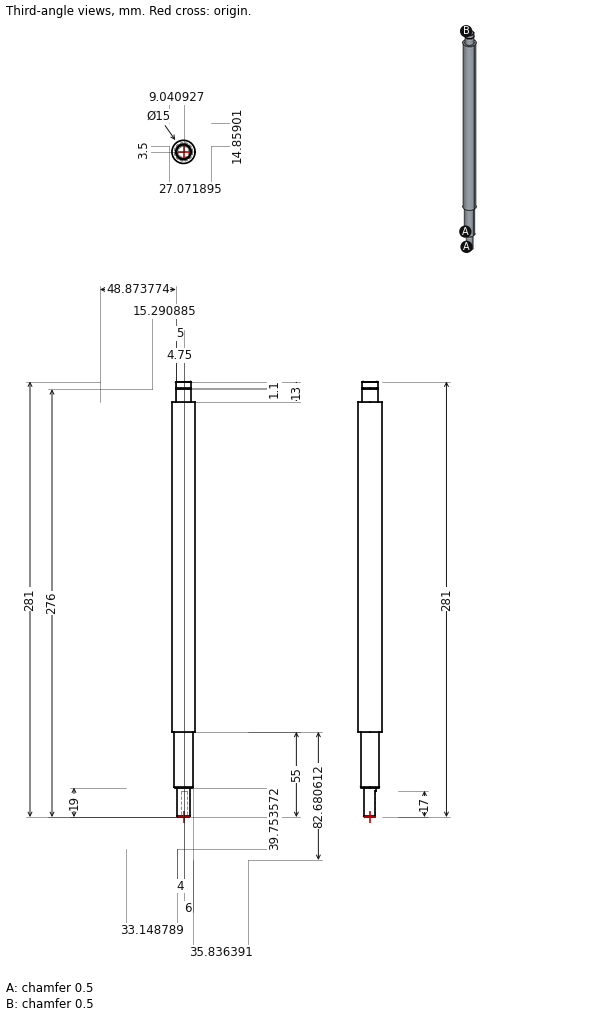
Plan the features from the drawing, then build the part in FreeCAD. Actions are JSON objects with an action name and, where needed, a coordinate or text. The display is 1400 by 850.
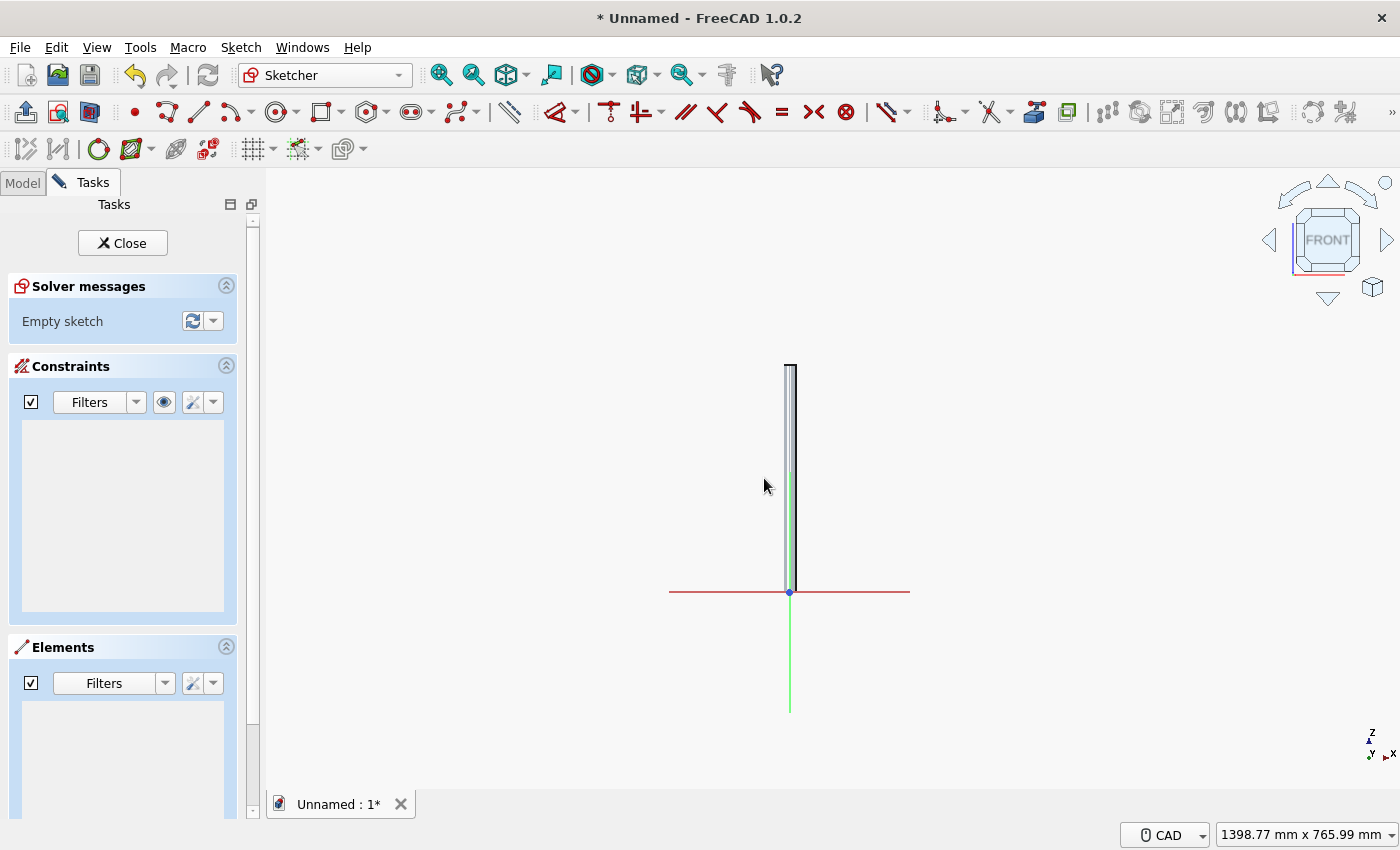
{"action": "scroll", "coordinate": [766, 363], "scroll_direction": "up", "scroll_amount": 14}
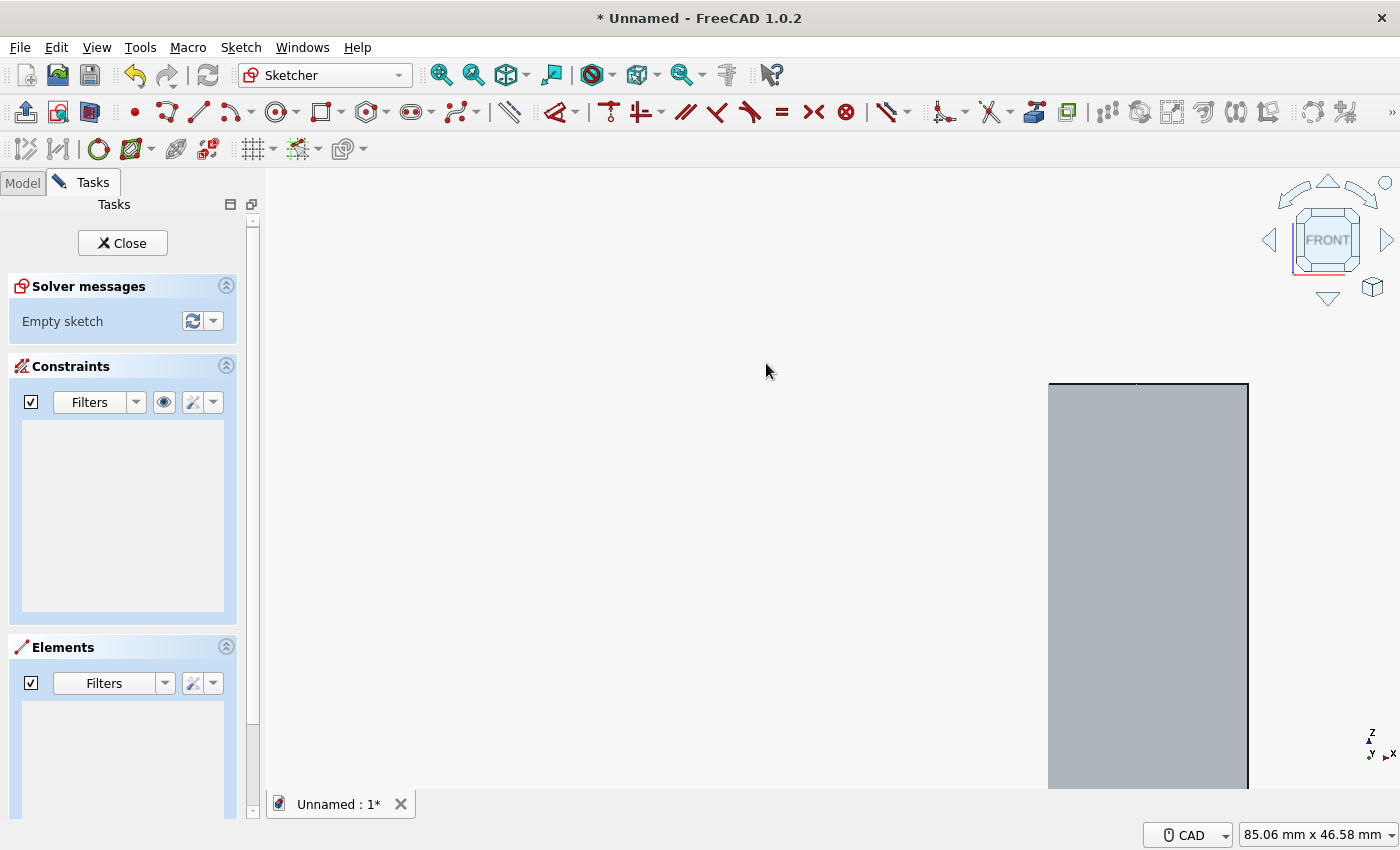
{"action": "left_click", "coordinate": [322, 112]}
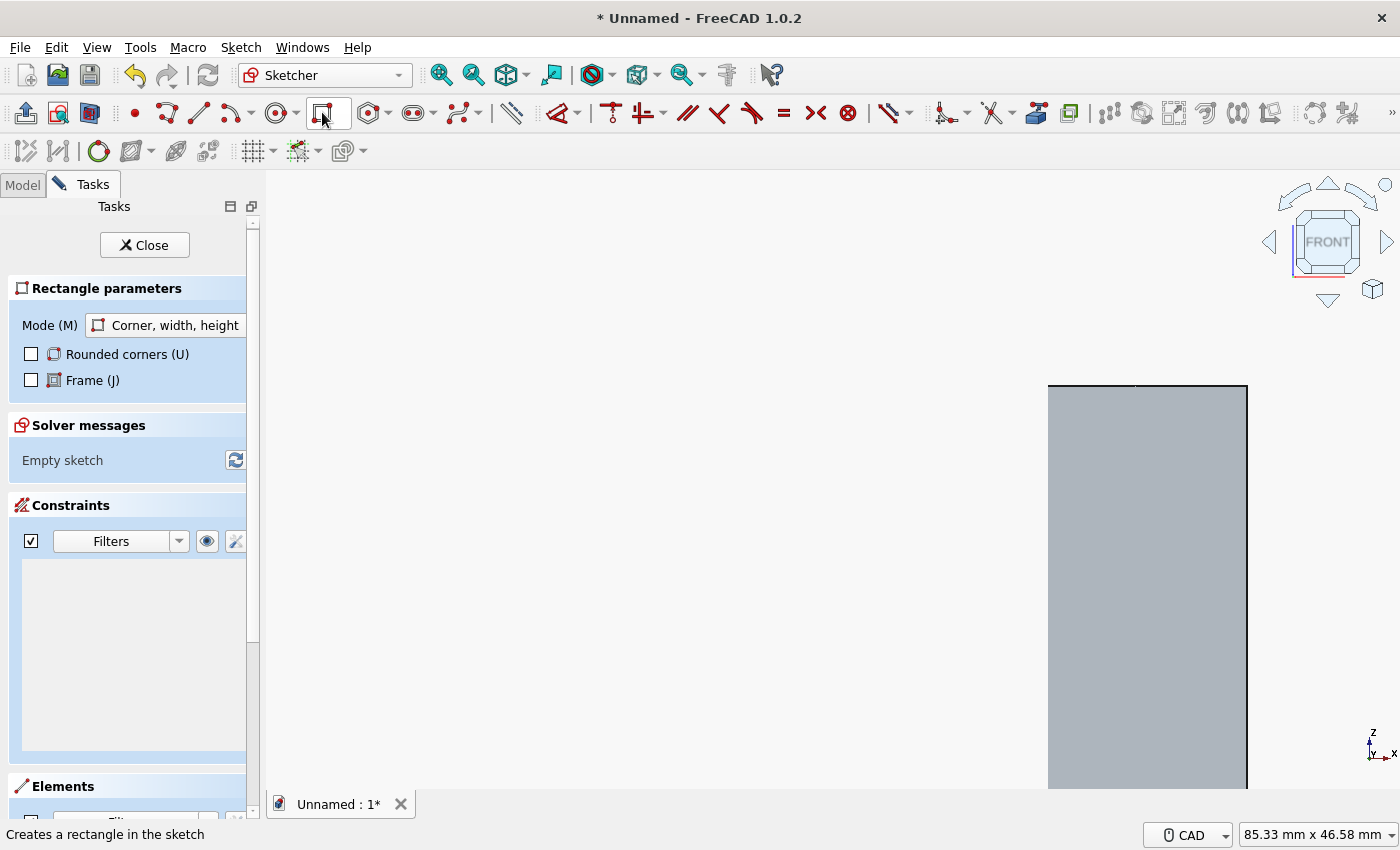
{"action": "left_click", "coordinate": [431, 386]}
{"action": "mouse_move", "coordinate": [1081, 558]}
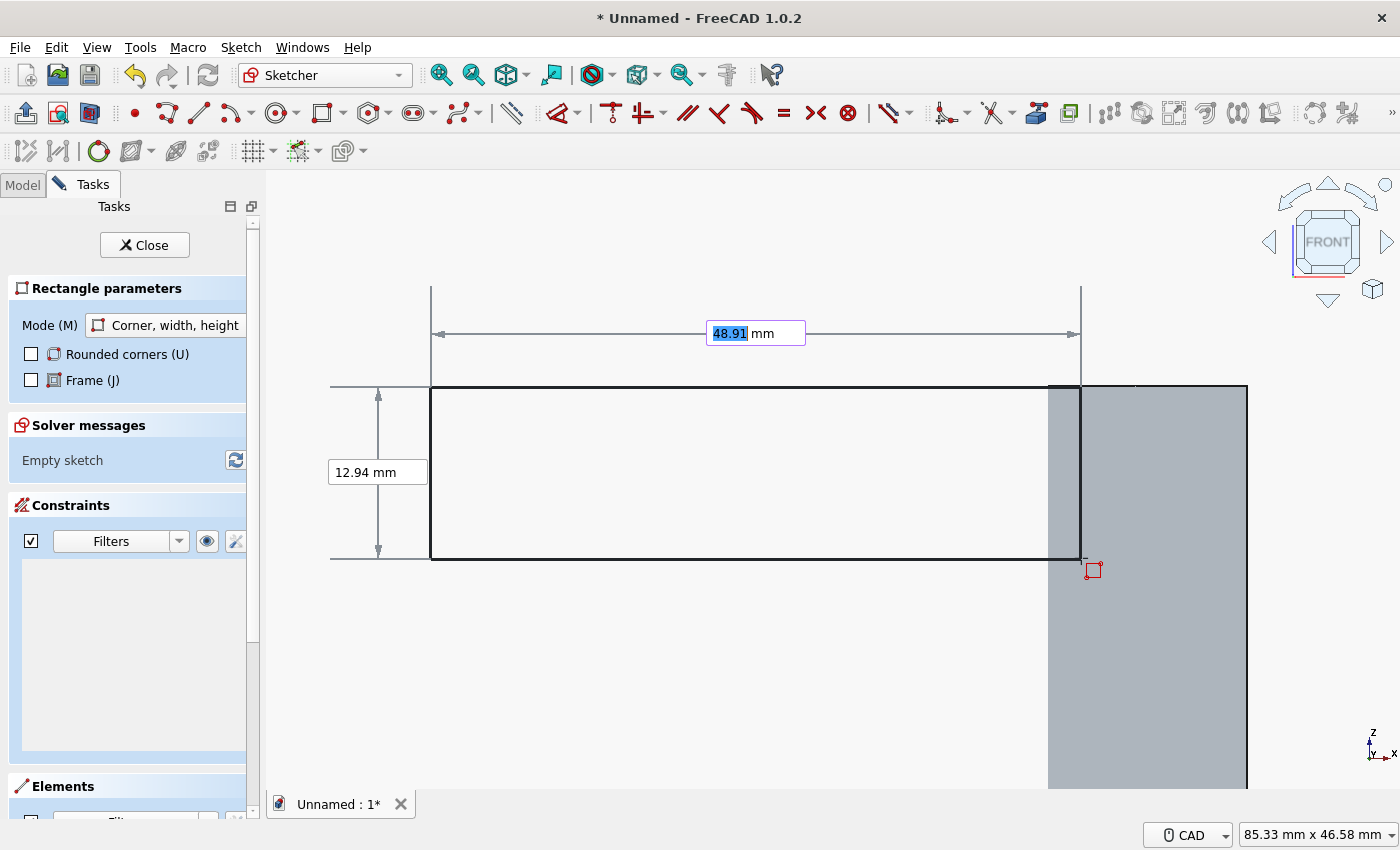
{"action": "type", "text": "48.873774"}
{"action": "key", "text": "Tab"}
{"action": "type", "text": "13"}
{"action": "key", "text": "Return"}
{"action": "key", "text": "Escape"}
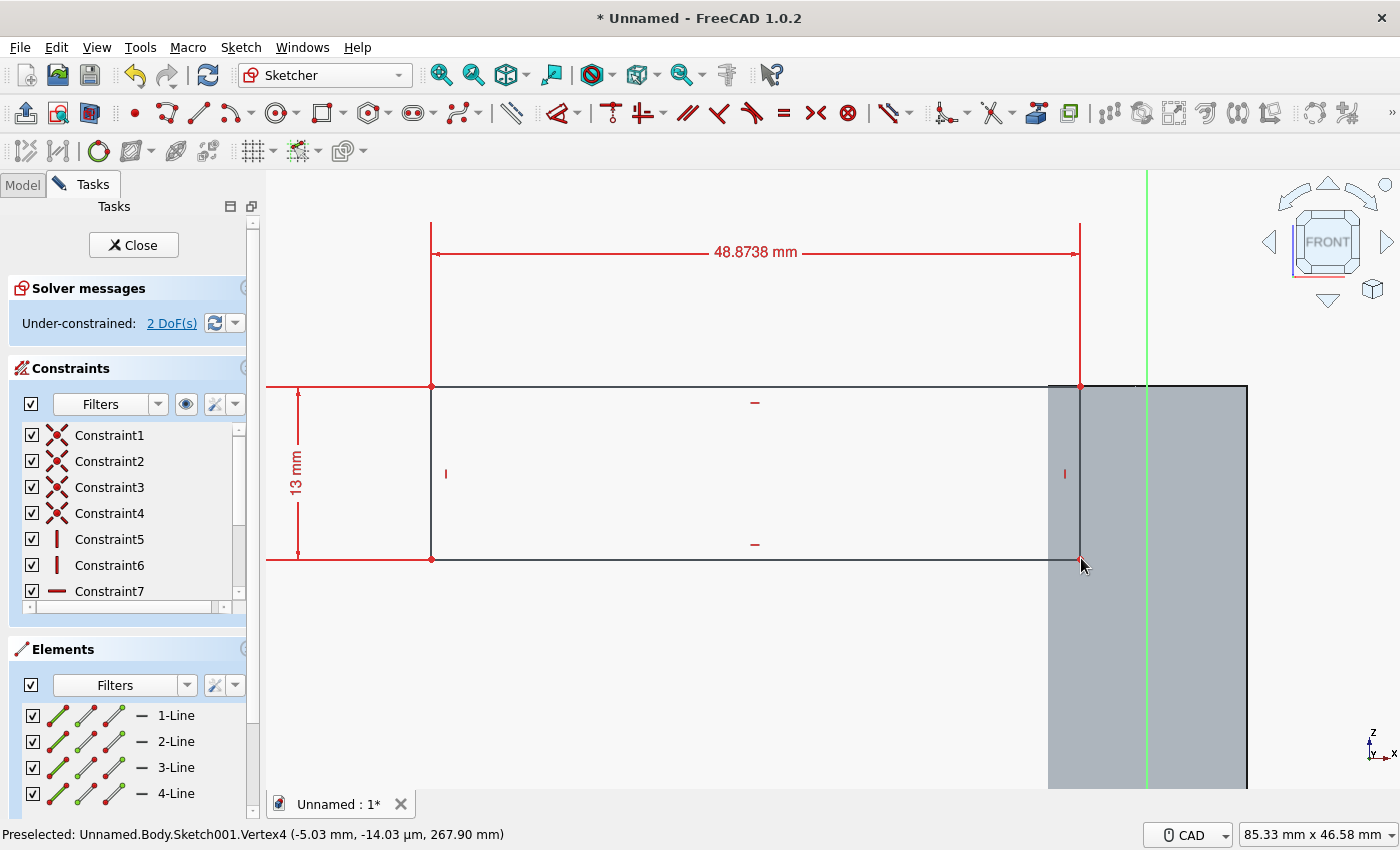
{"action": "left_click", "coordinate": [558, 114]}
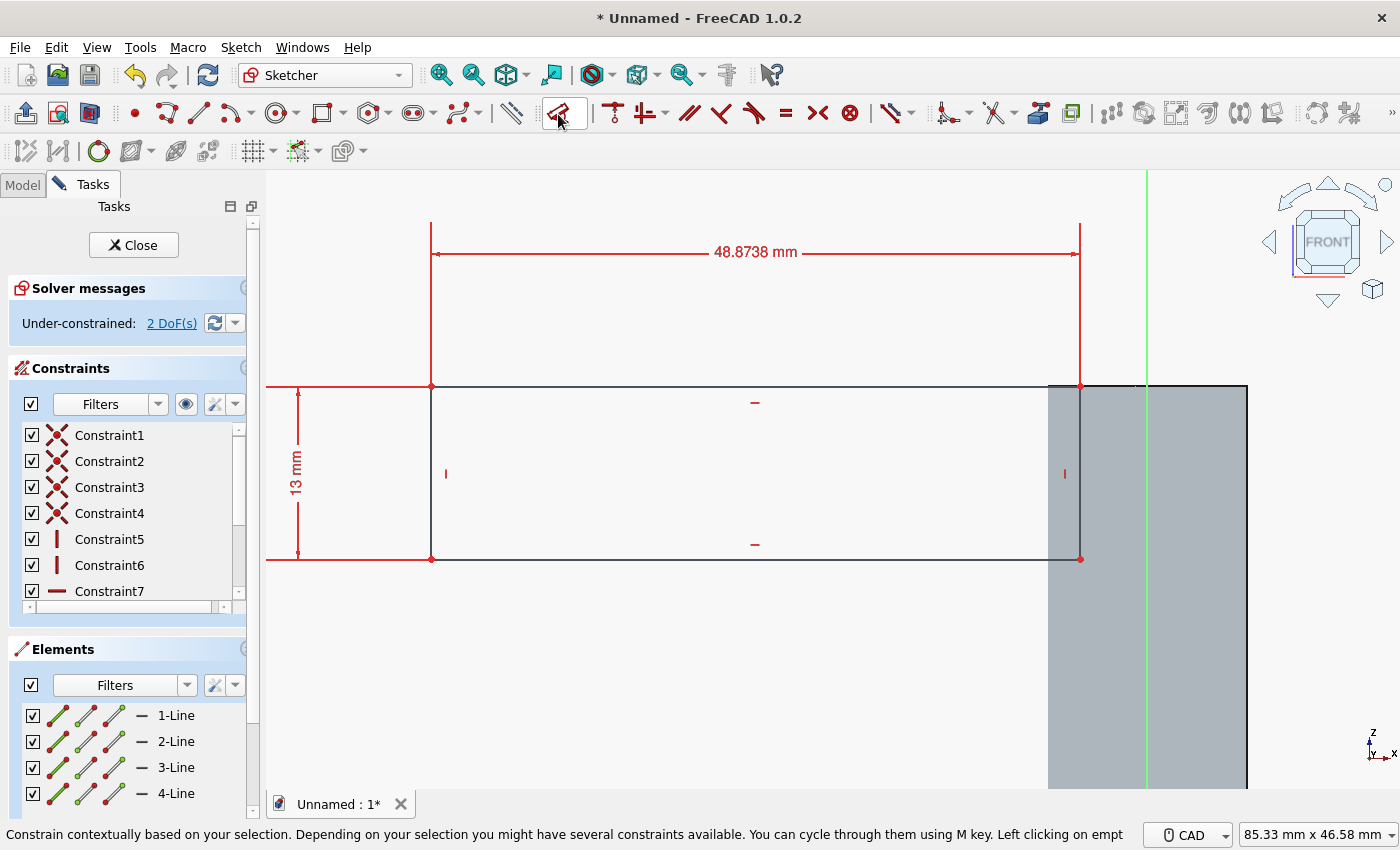
{"action": "left_click", "coordinate": [1080, 560]}
{"action": "left_click", "coordinate": [1114, 526]}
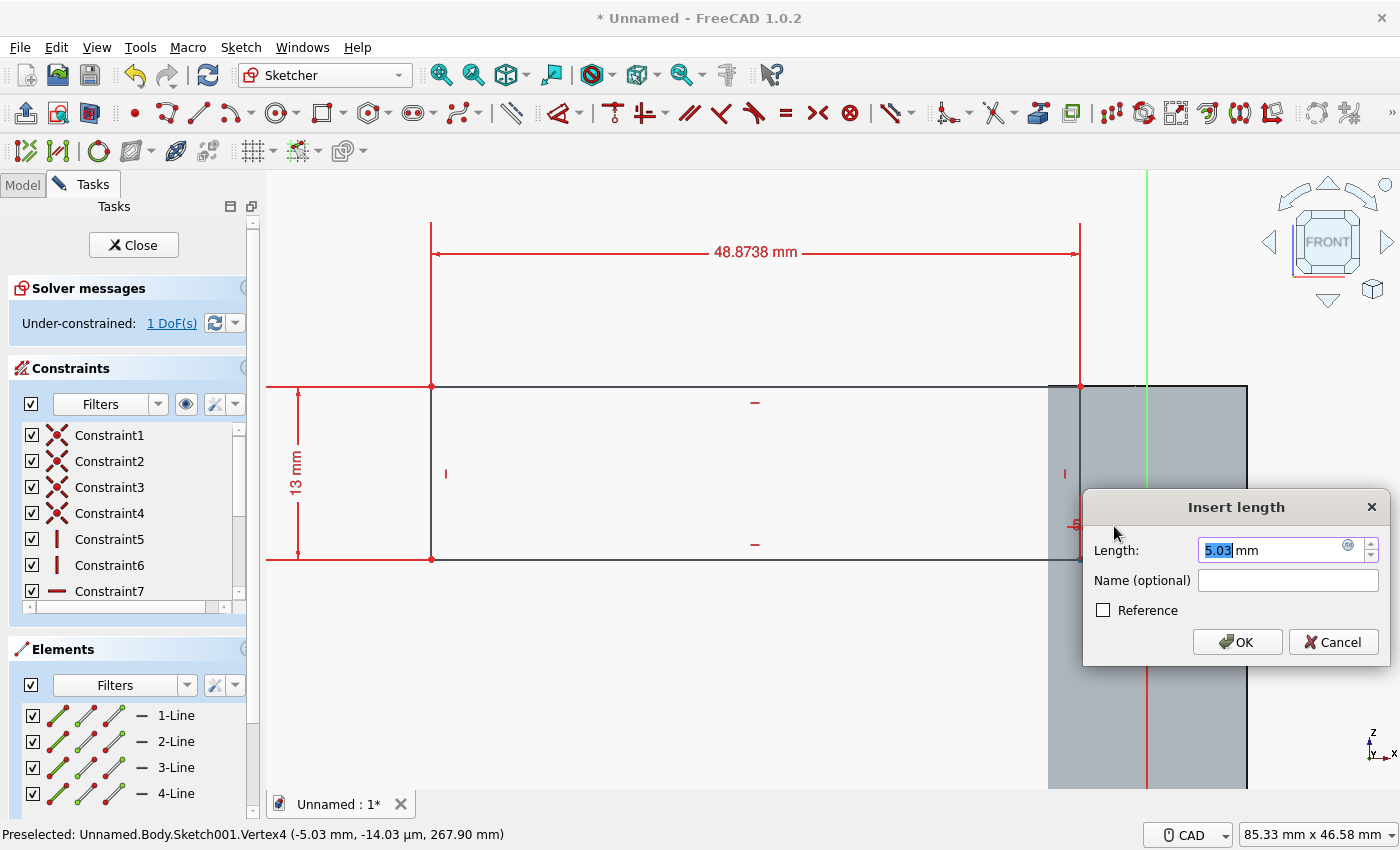
{"action": "type", "text": "5"}
{"action": "key", "text": "Return"}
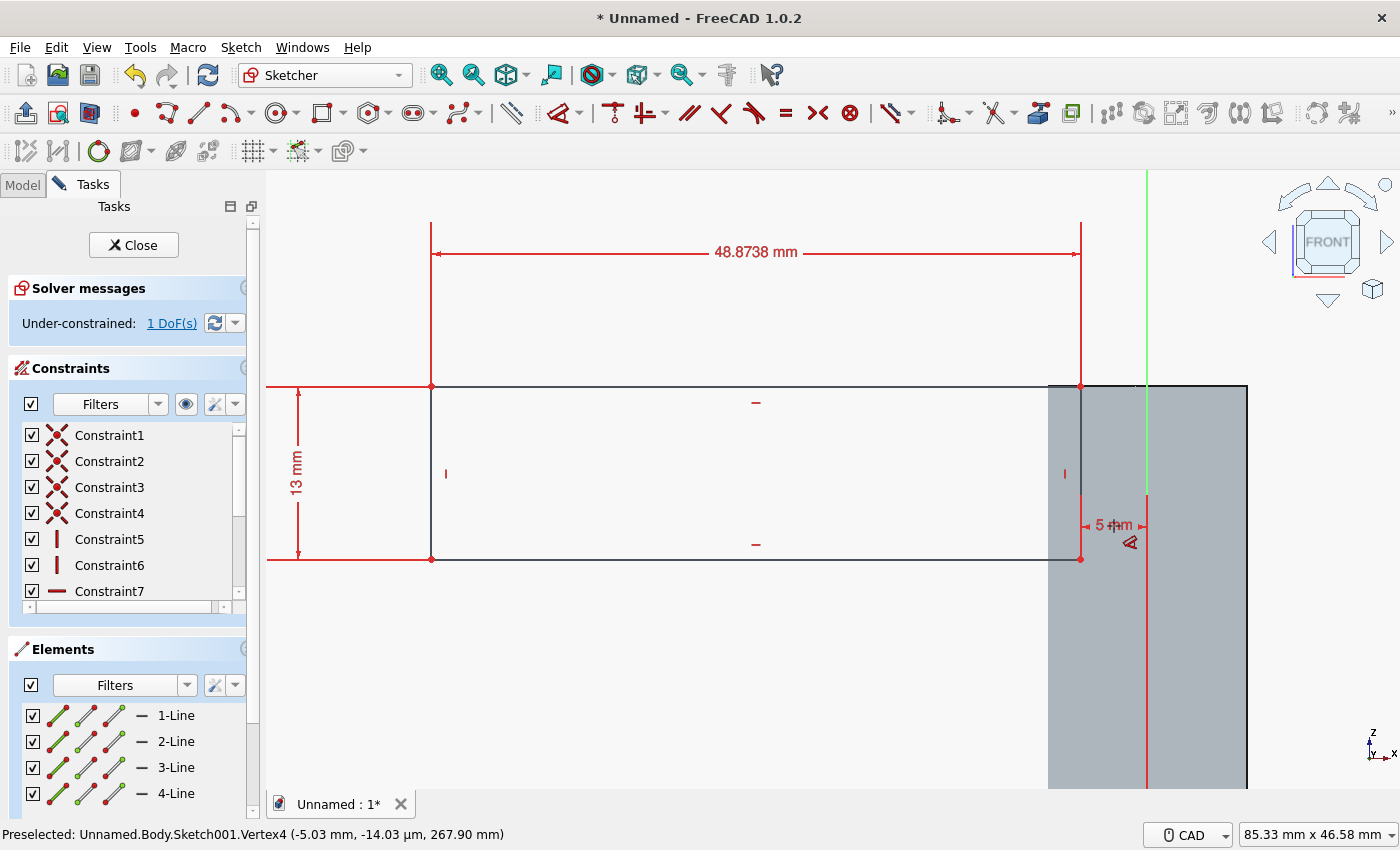
{"action": "left_click", "coordinate": [431, 387]}
{"action": "left_click", "coordinate": [1181, 574]}